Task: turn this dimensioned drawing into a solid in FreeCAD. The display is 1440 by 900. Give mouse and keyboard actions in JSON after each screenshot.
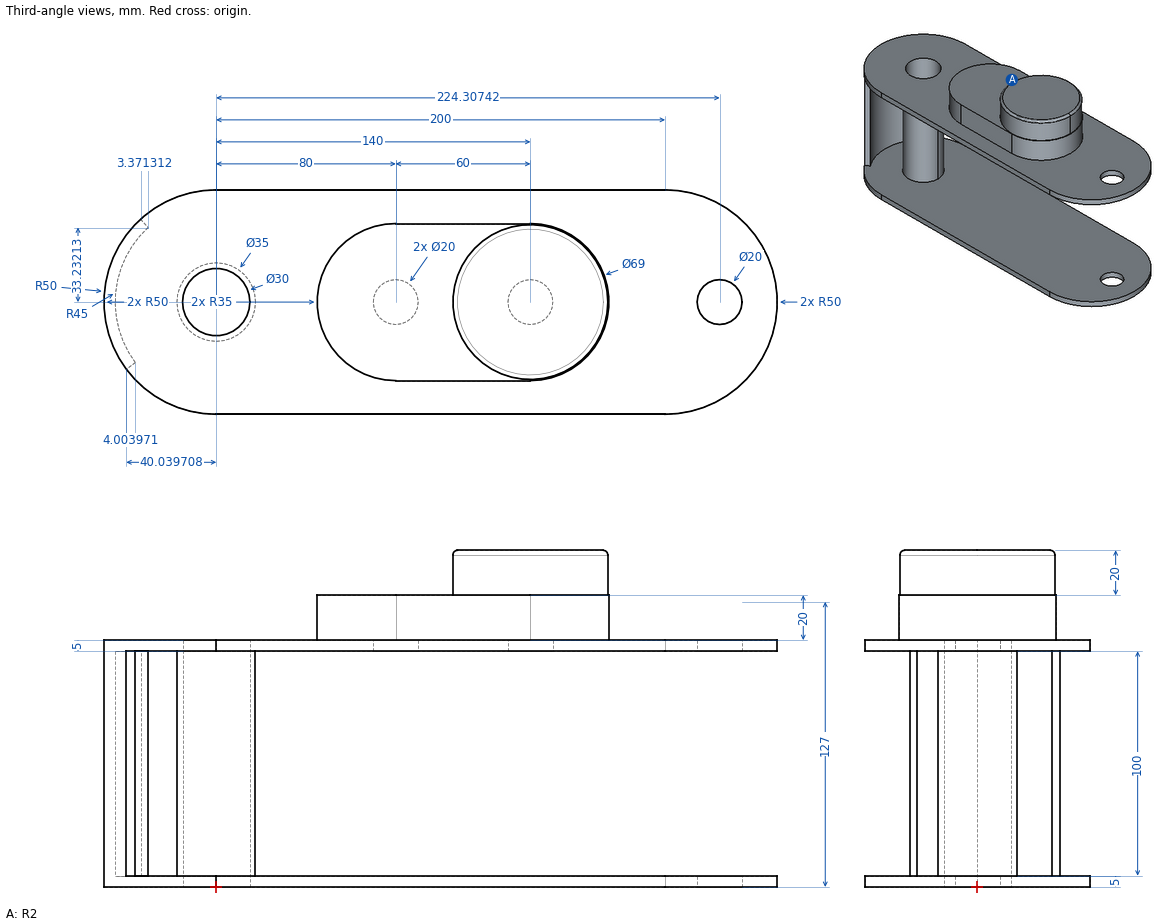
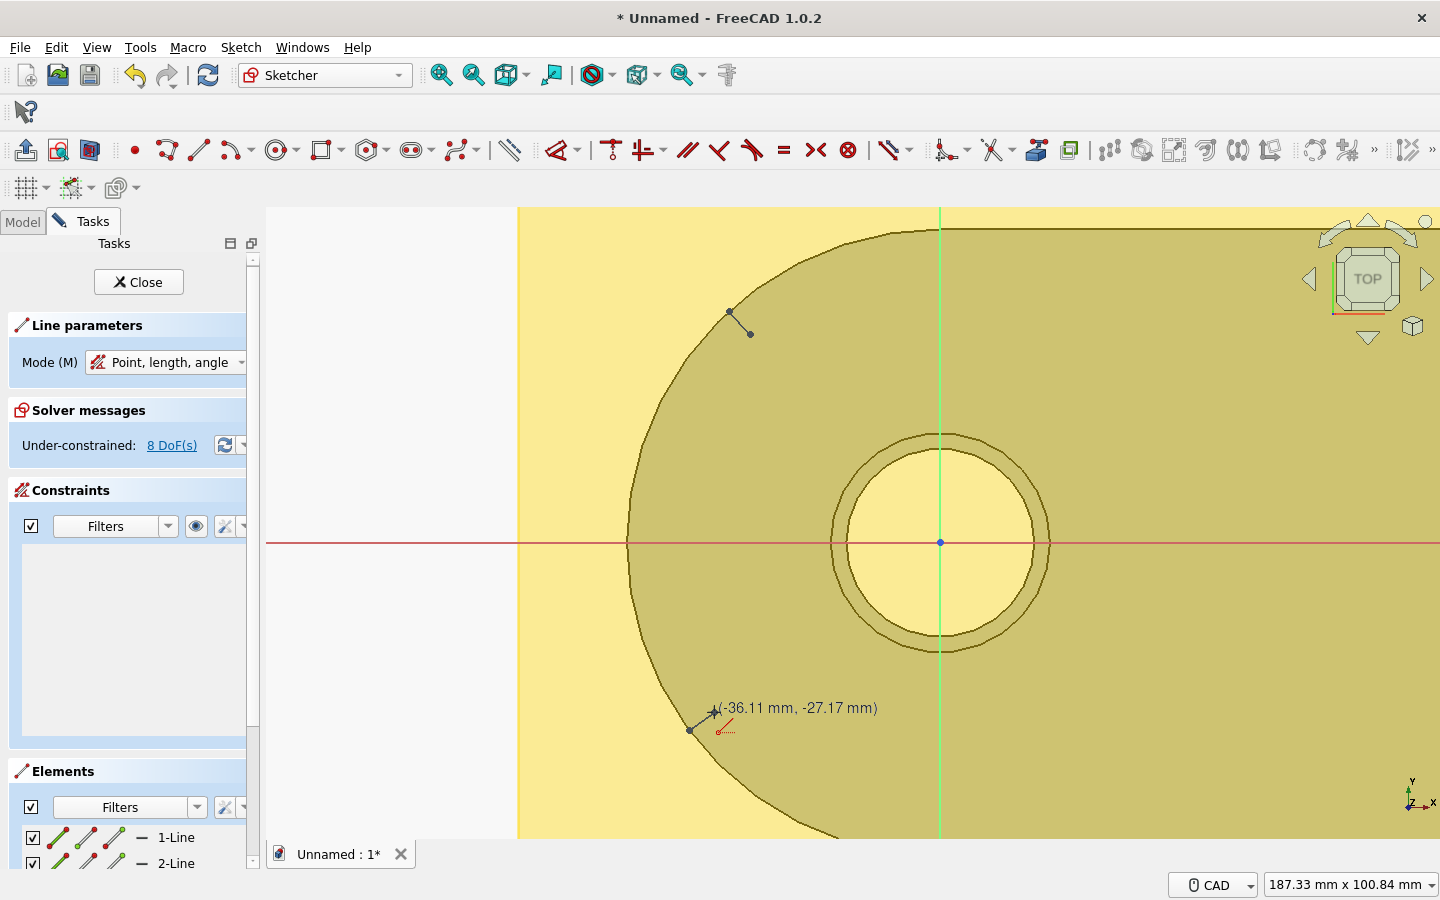
{"action": "left_click", "coordinate": [254, 150]}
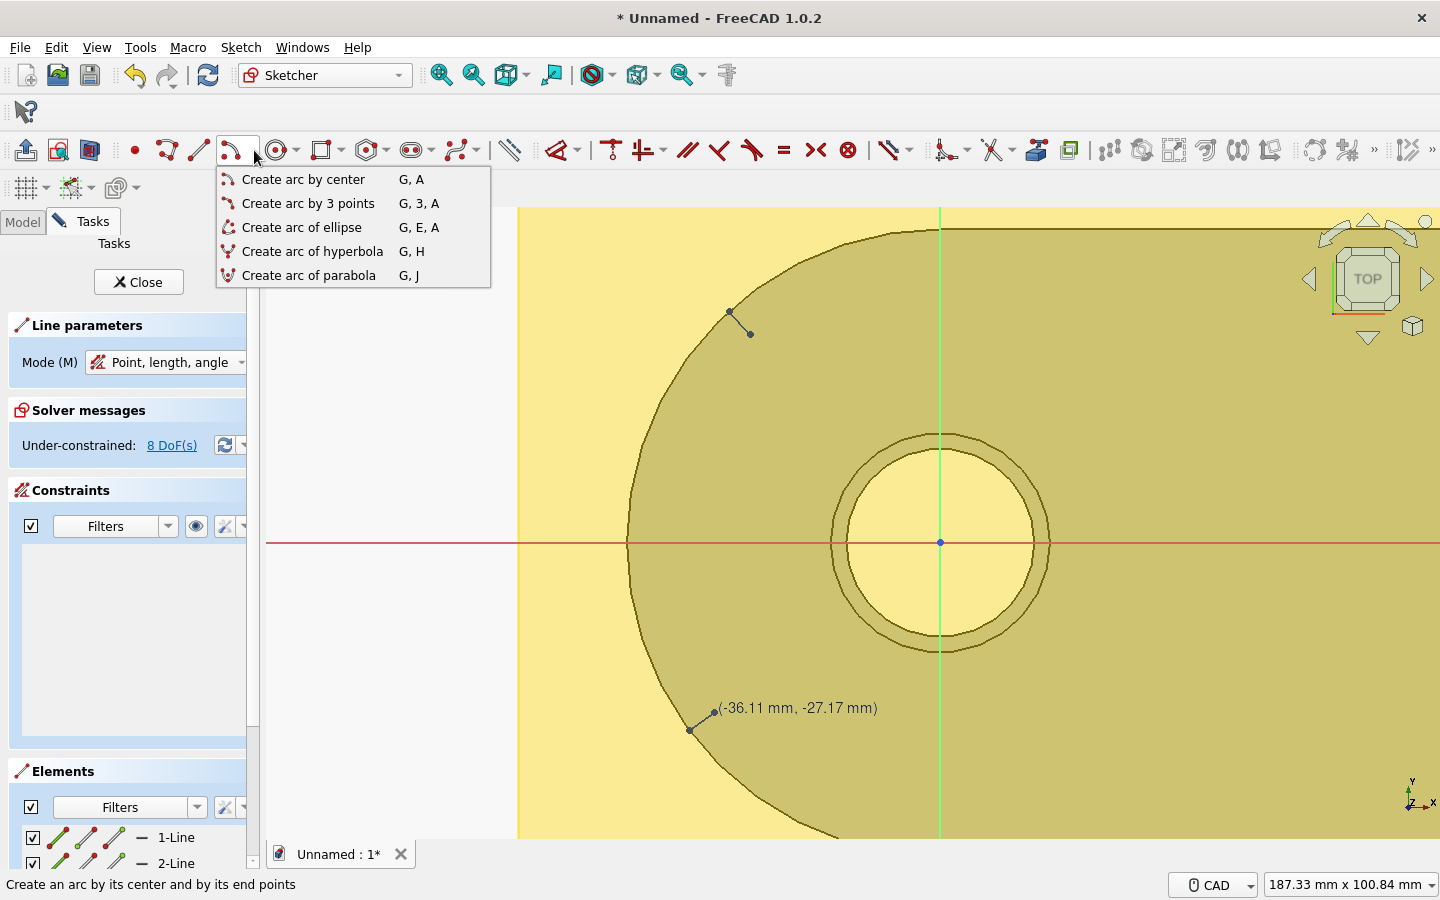
{"action": "left_click", "coordinate": [354, 203]}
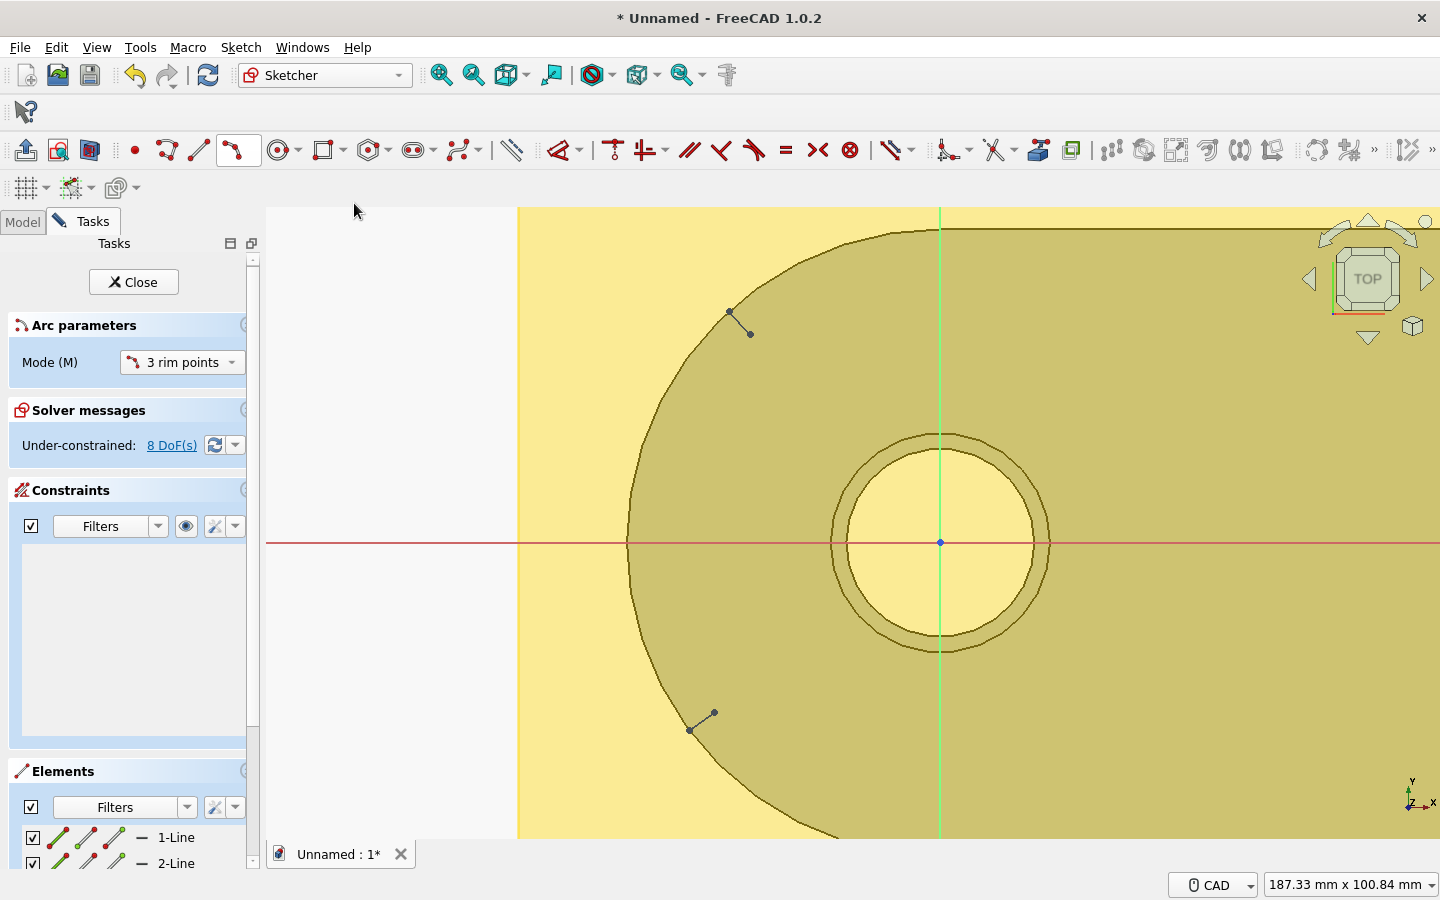
{"action": "left_click", "coordinate": [729, 312]}
{"action": "left_click", "coordinate": [689, 731]}
{"action": "left_click", "coordinate": [628, 513]}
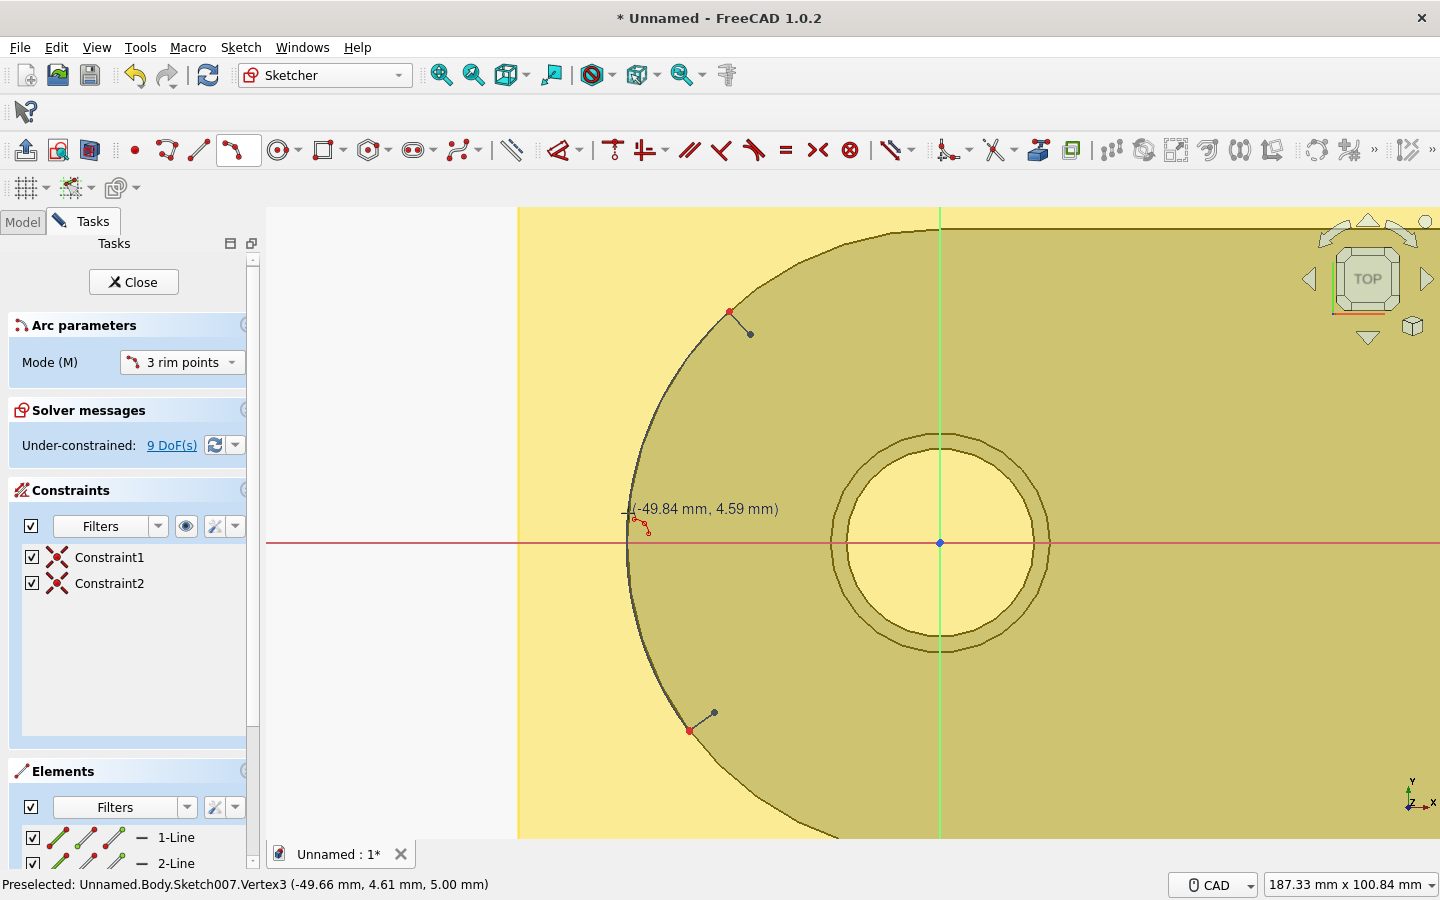
{"action": "left_click", "coordinate": [714, 713]}
{"action": "left_click", "coordinate": [750, 335]}
{"action": "left_click", "coordinate": [660, 516]}
{"action": "key", "text": "Escape"}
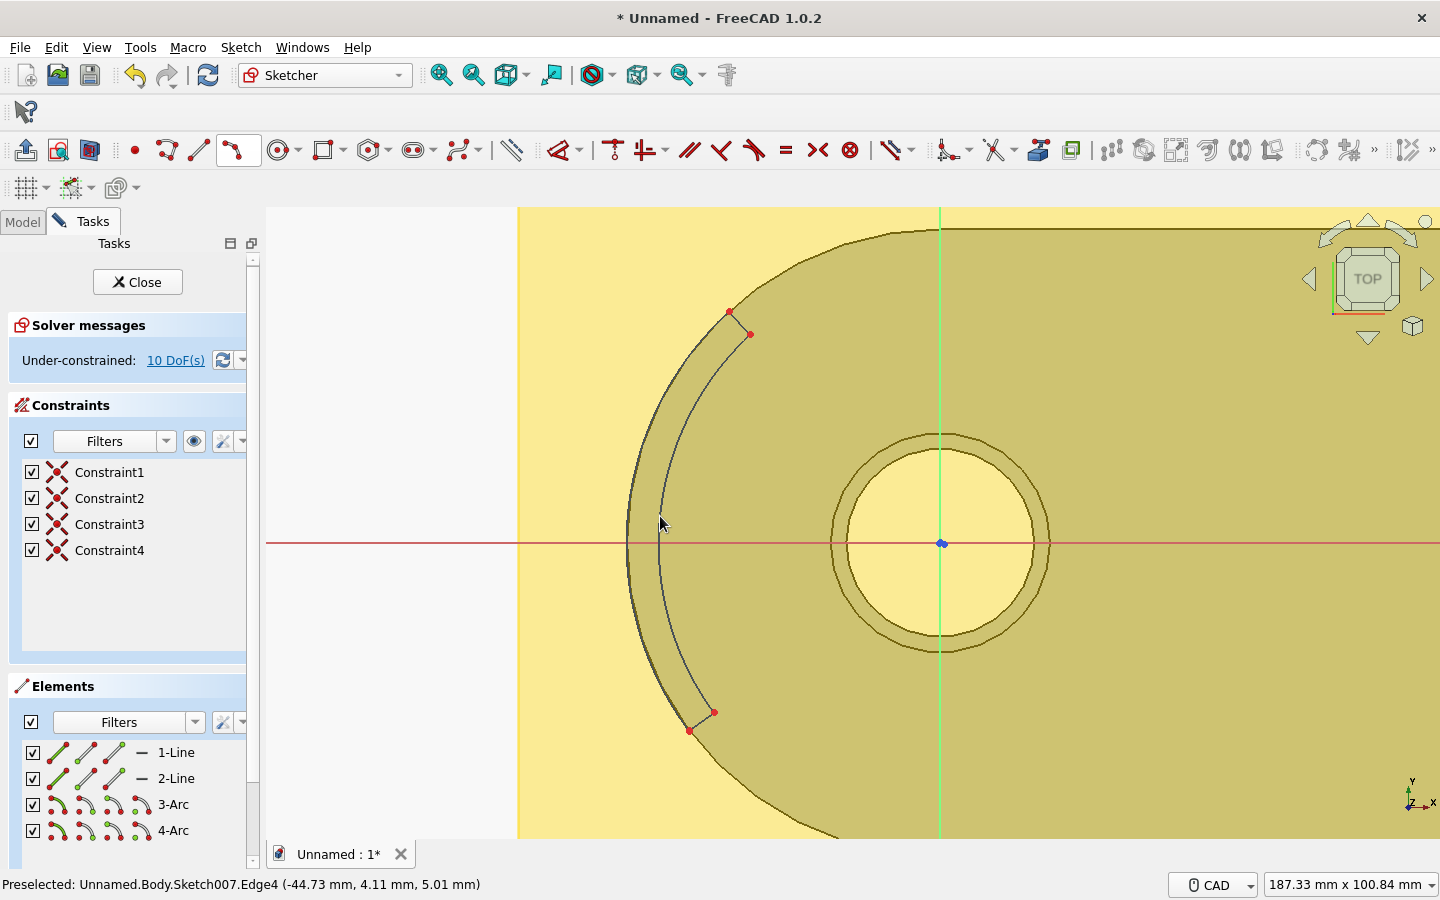
{"action": "left_click", "coordinate": [650, 424]}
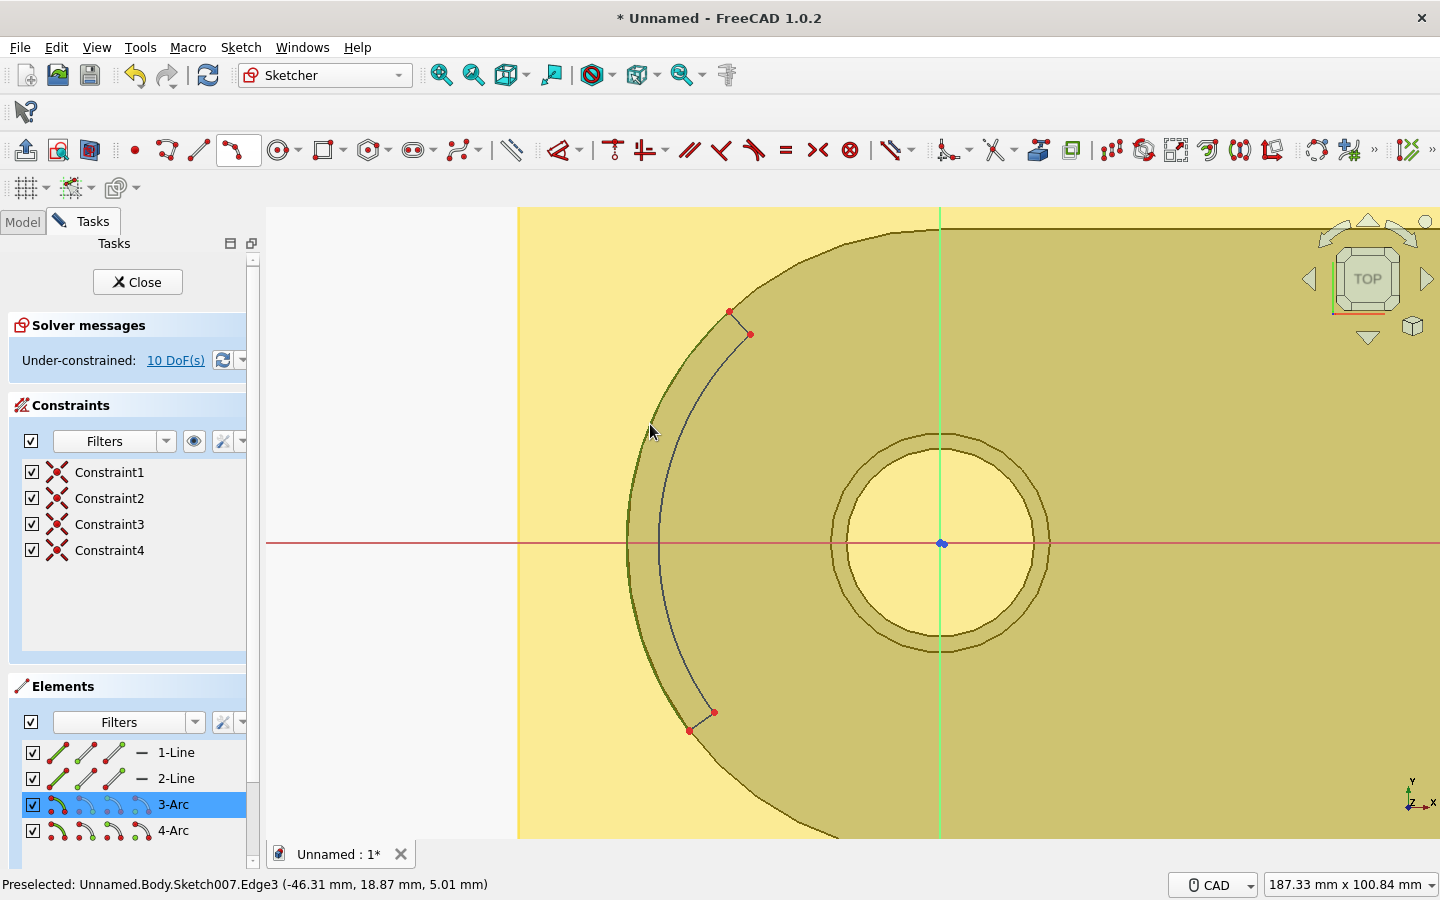
{"action": "left_click", "coordinate": [680, 437]}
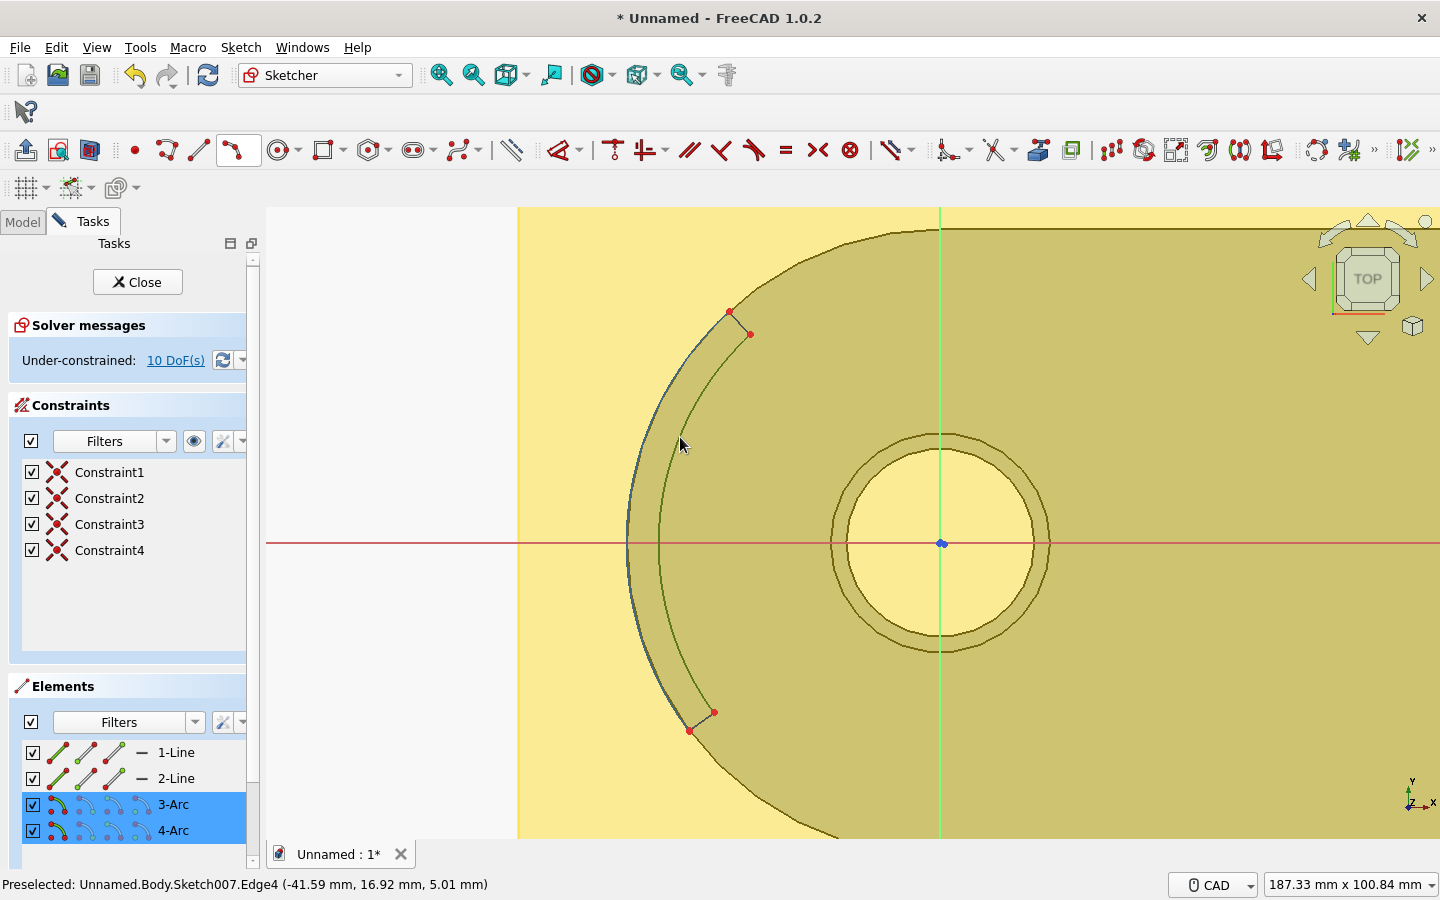
{"action": "left_click", "coordinate": [614, 150]}